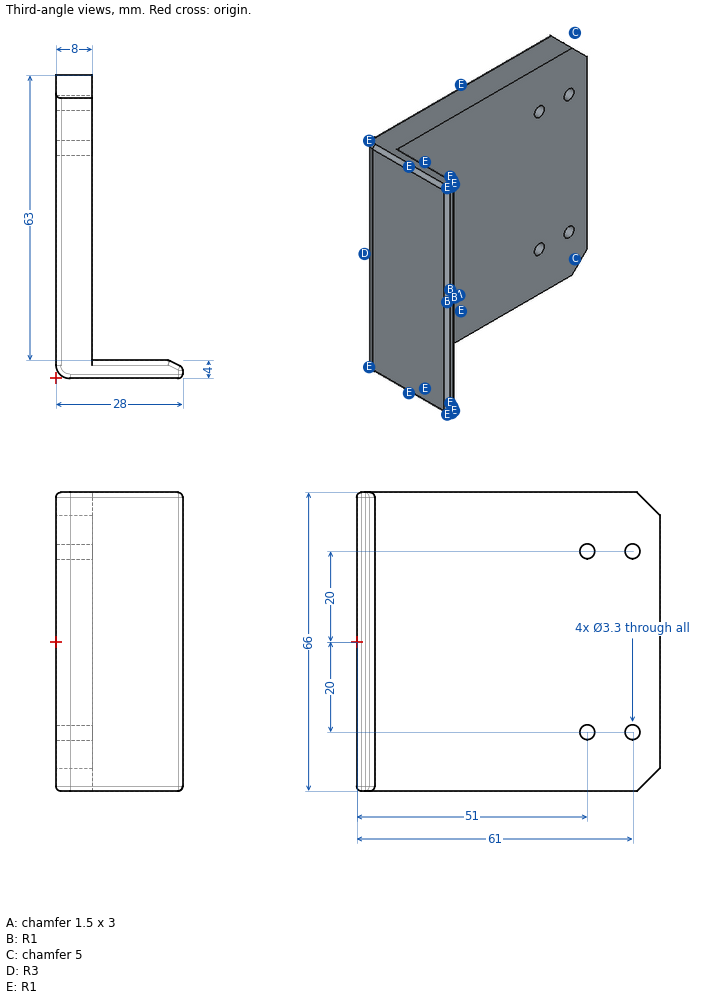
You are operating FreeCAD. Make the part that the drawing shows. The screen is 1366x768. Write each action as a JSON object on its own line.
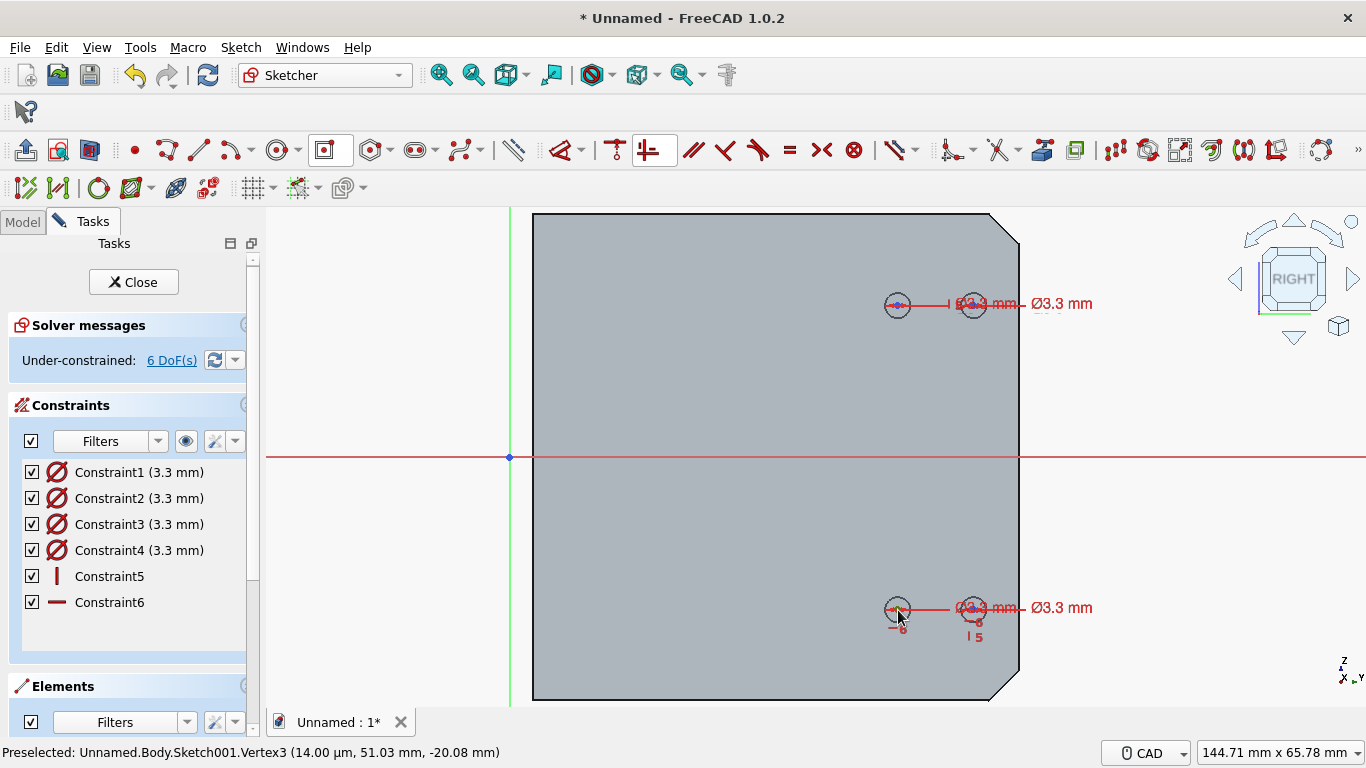
{"action": "left_click", "coordinate": [898, 306]}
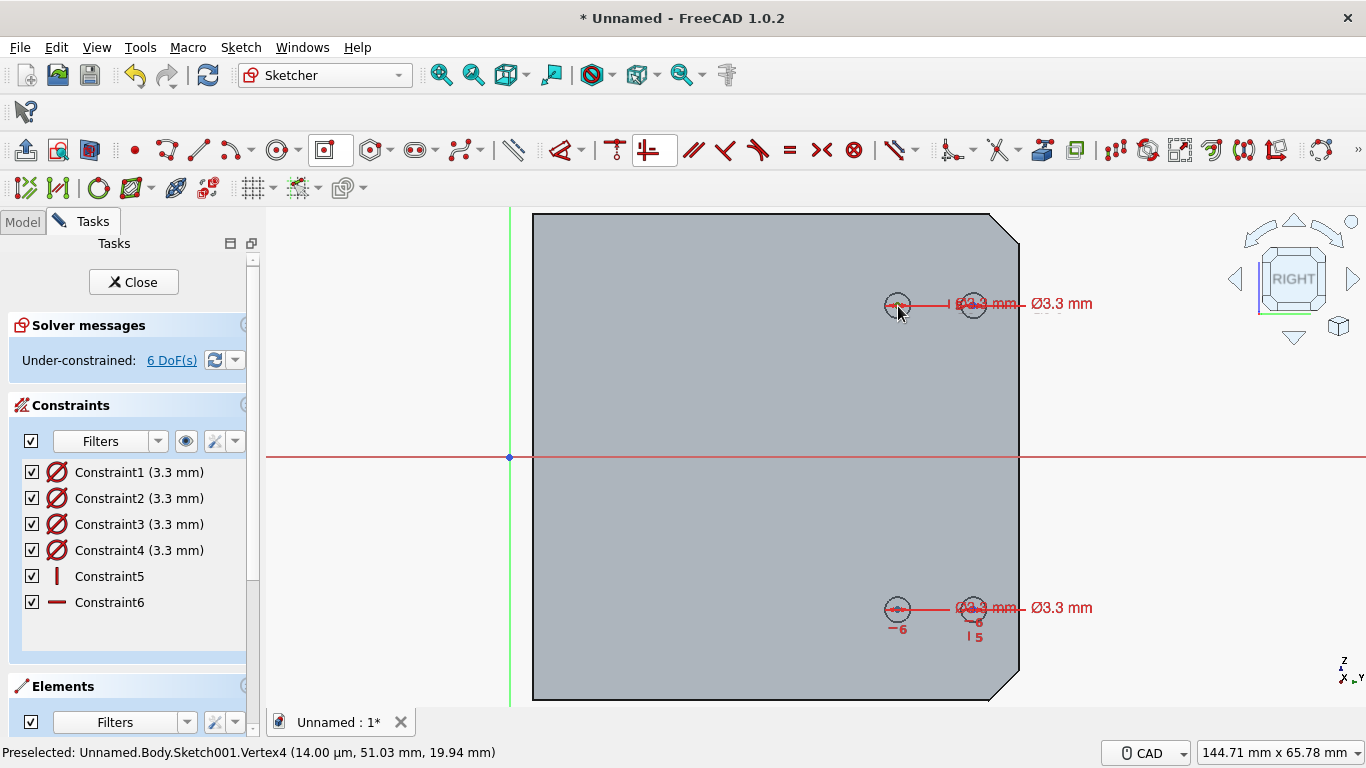
{"action": "left_click", "coordinate": [672, 150]}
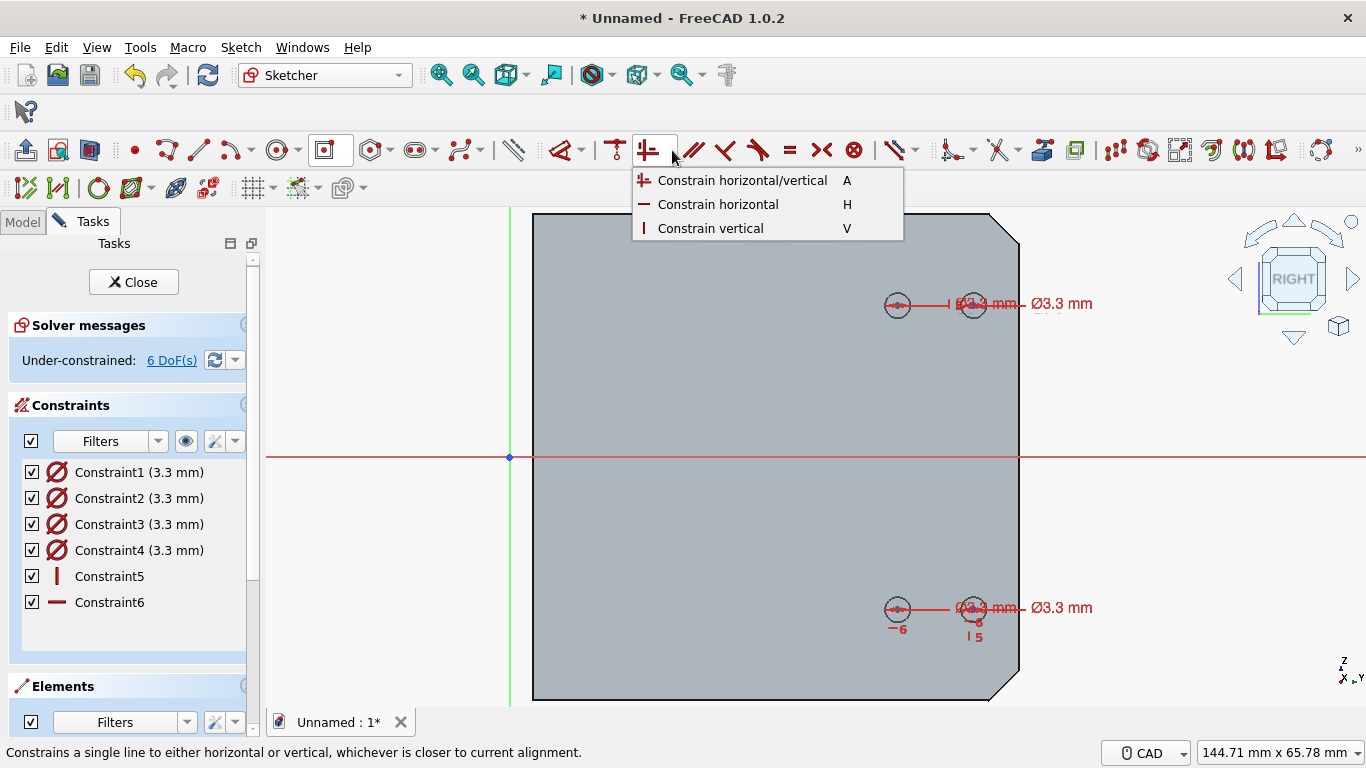
{"action": "left_click", "coordinate": [768, 228]}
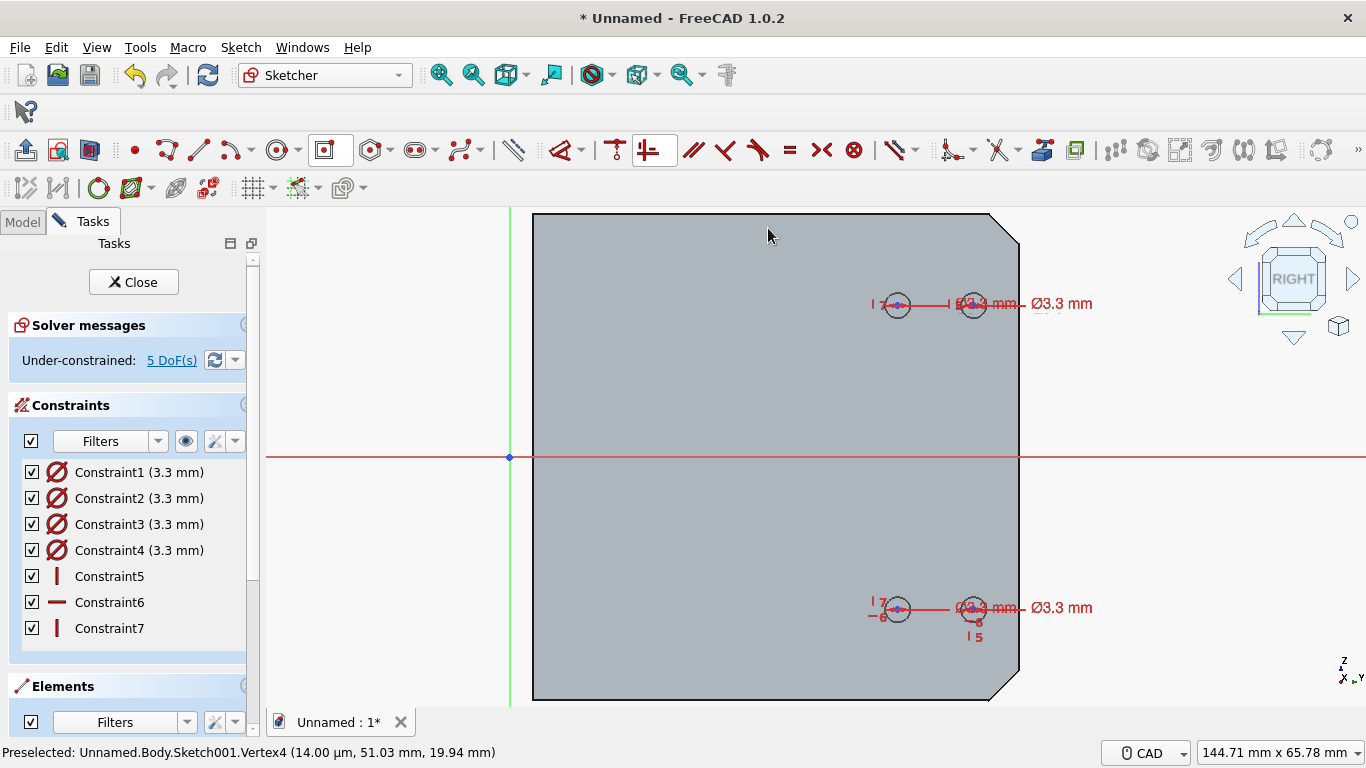
{"action": "left_click", "coordinate": [974, 306]}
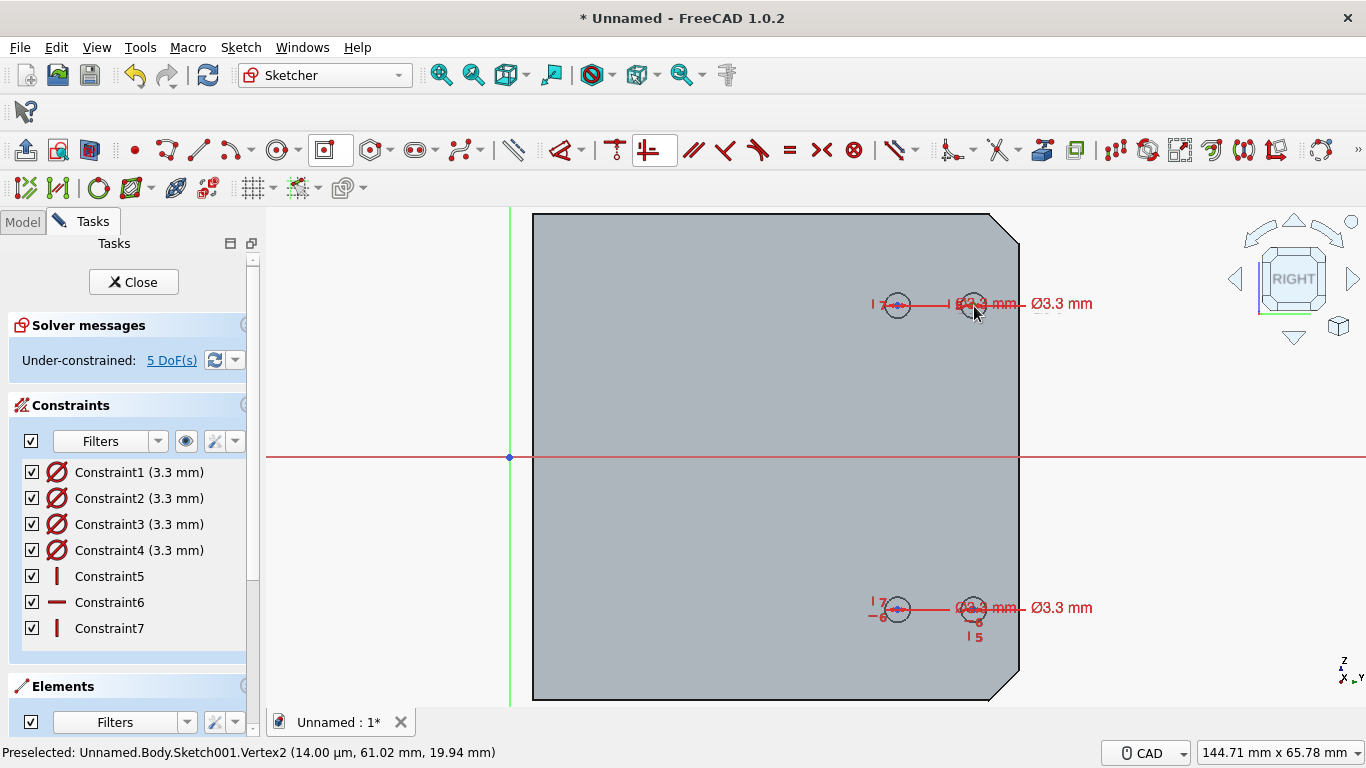
{"action": "left_click", "coordinate": [898, 306]}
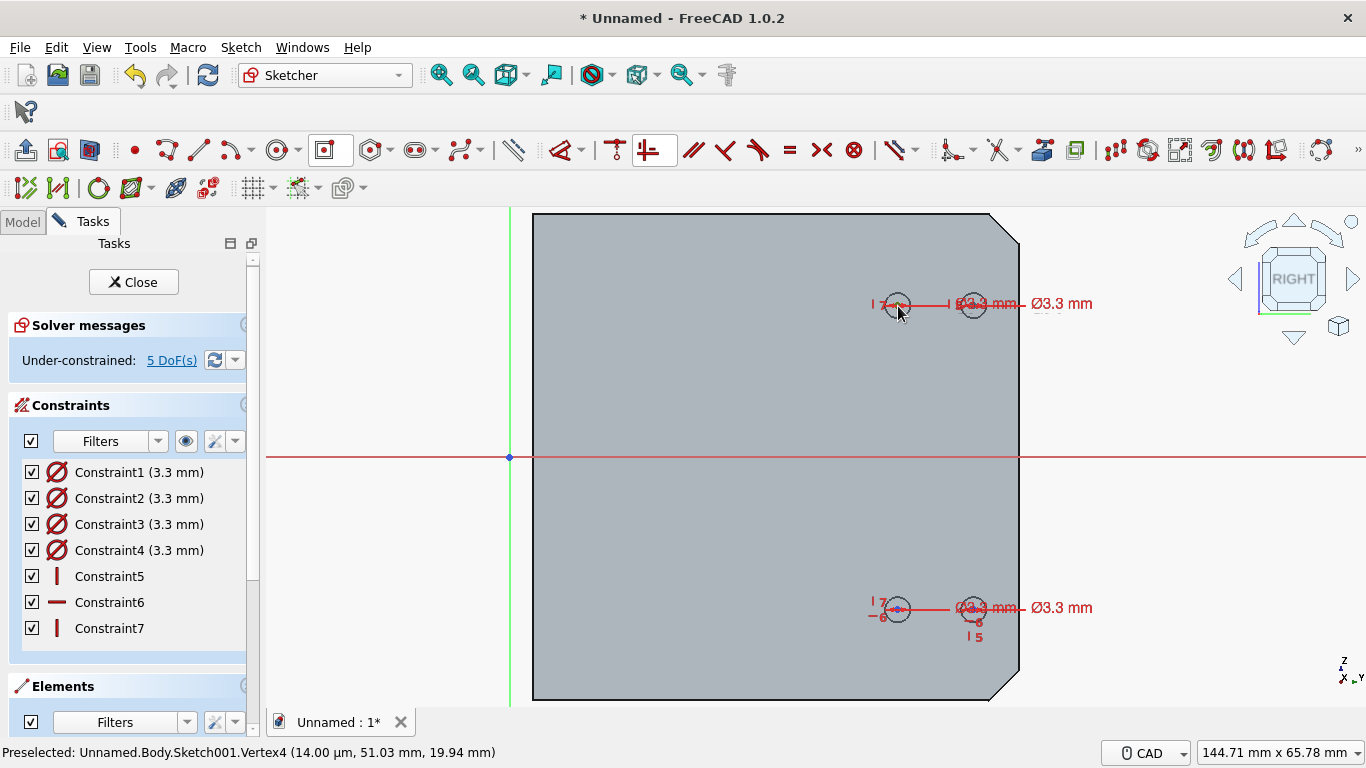
{"action": "key", "text": "h"}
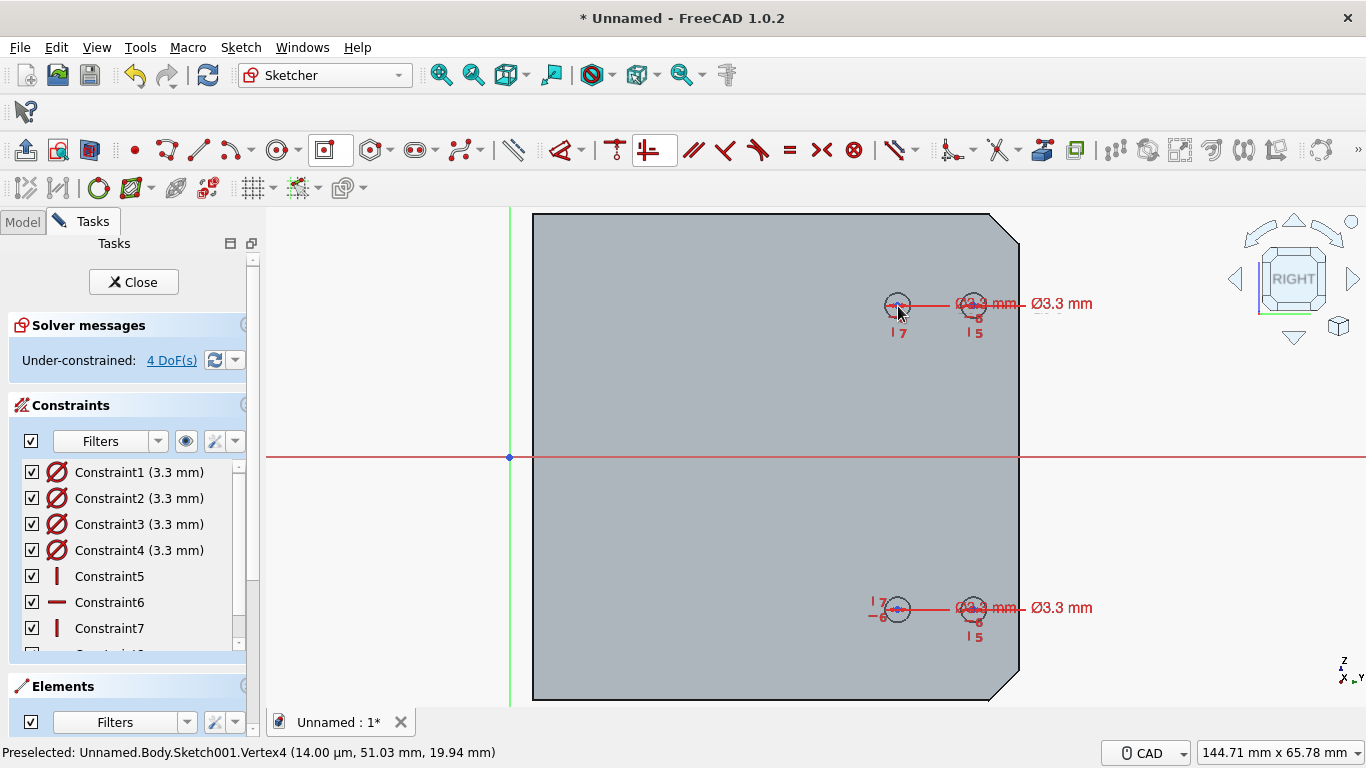
{"action": "key", "text": "d"}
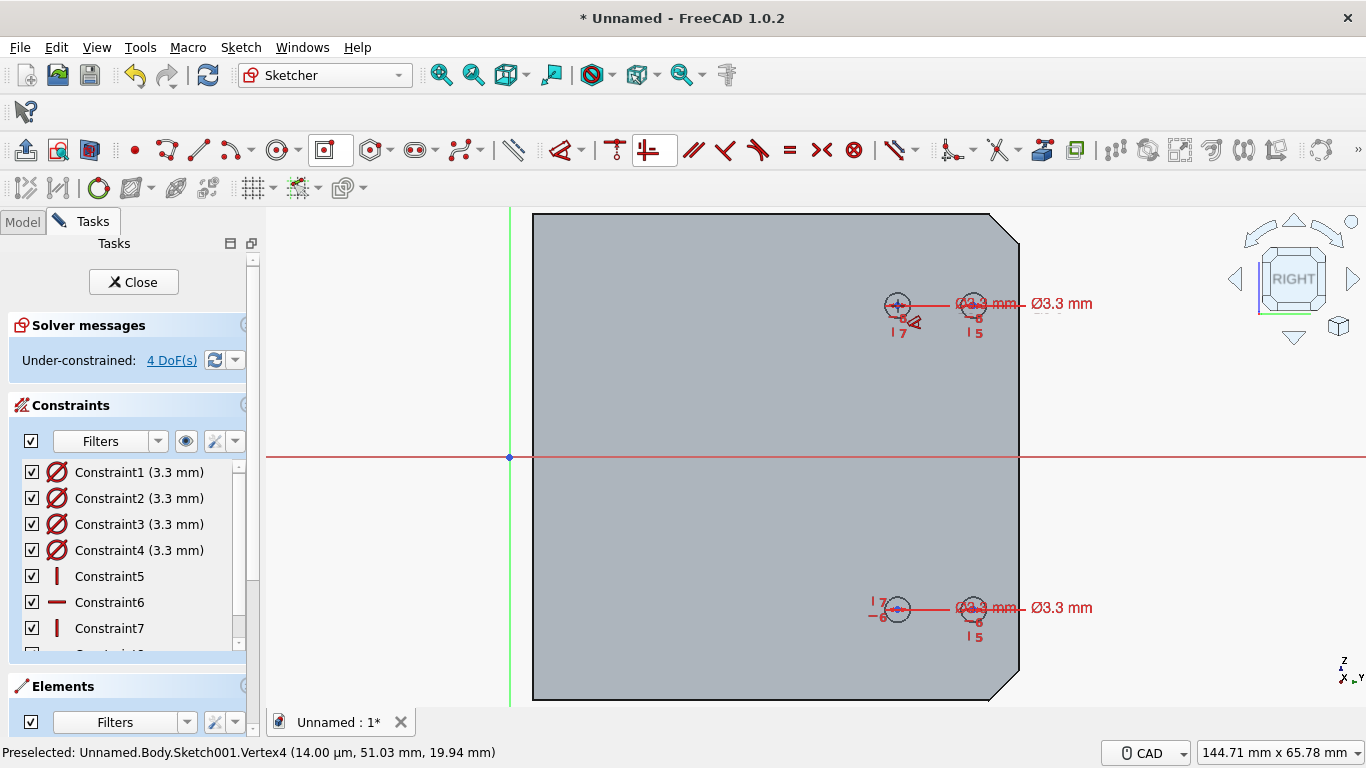
{"action": "left_click", "coordinate": [974, 610]}
{"action": "left_click", "coordinate": [742, 644]}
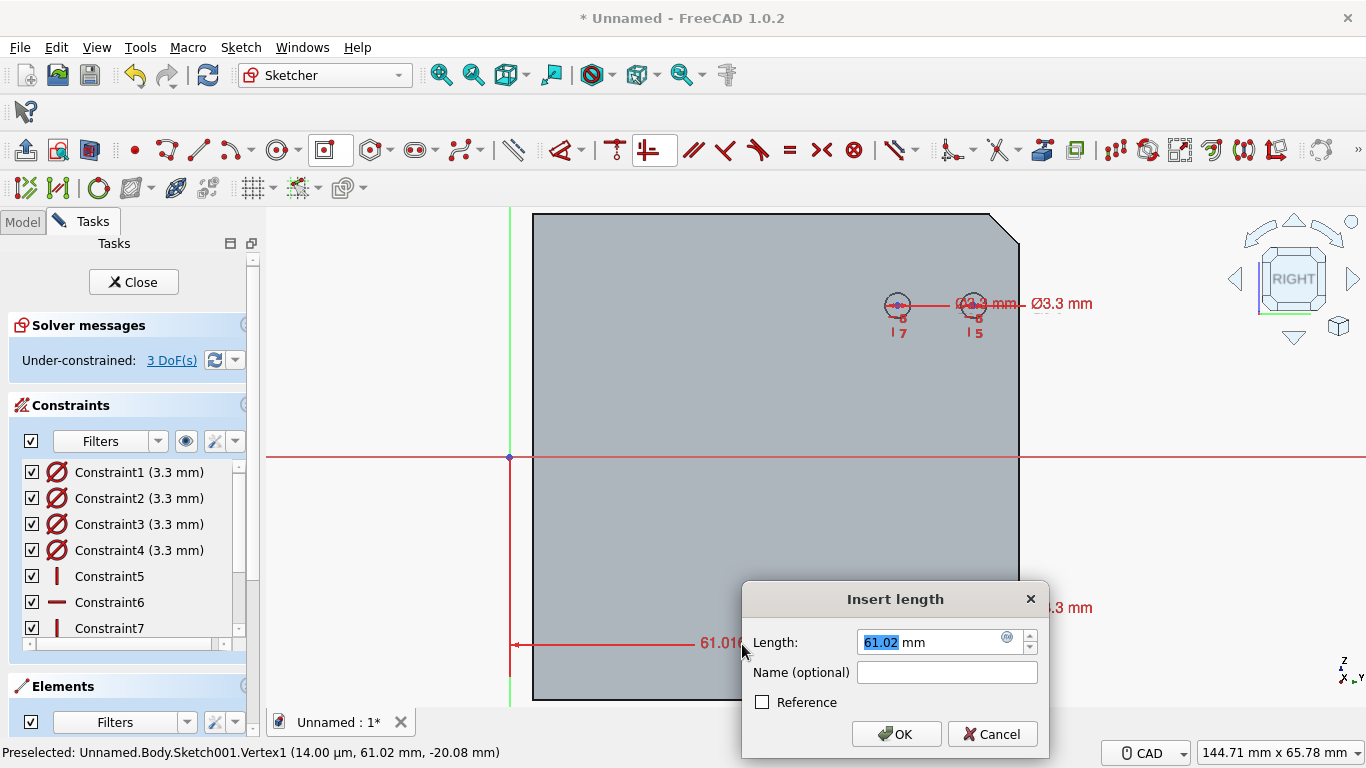
{"action": "type", "text": "61"}
{"action": "key", "text": "Return"}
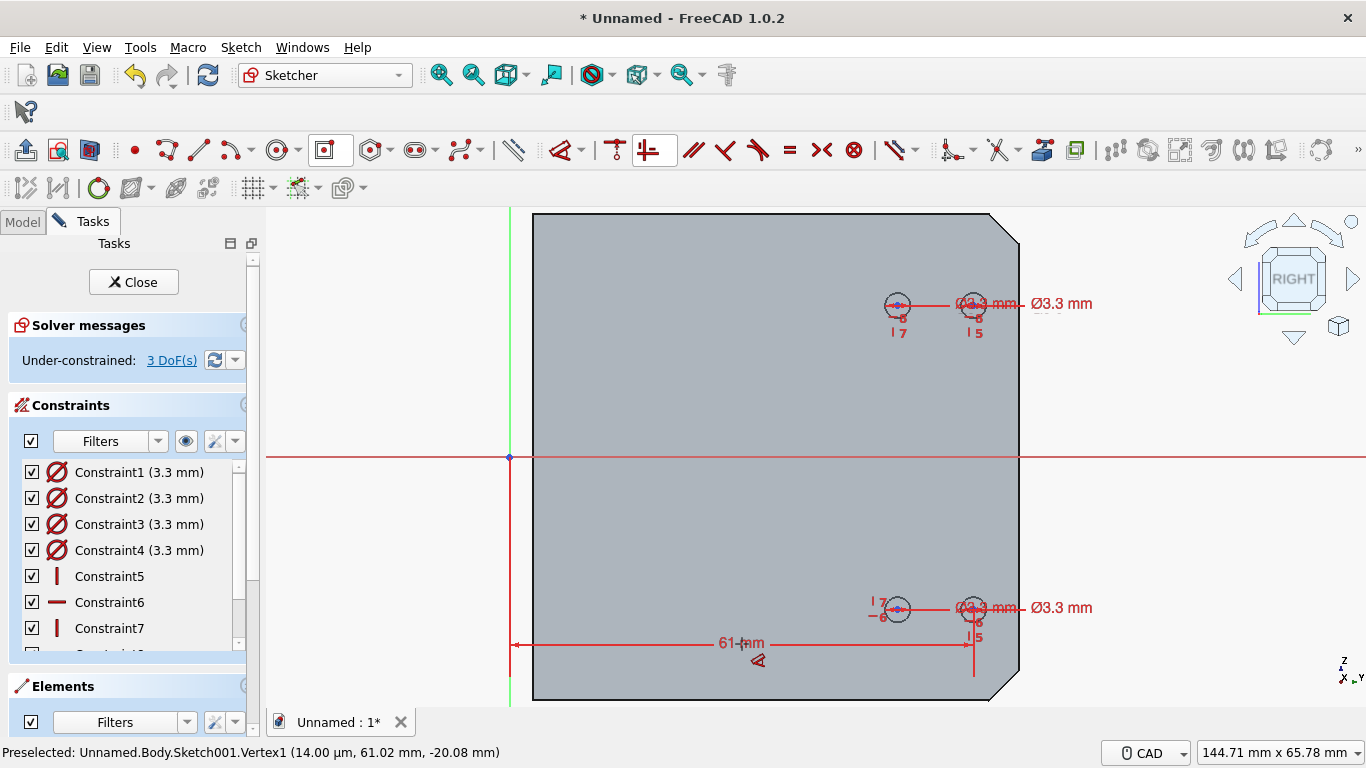
{"action": "left_click", "coordinate": [974, 610]}
{"action": "left_click", "coordinate": [476, 534]}